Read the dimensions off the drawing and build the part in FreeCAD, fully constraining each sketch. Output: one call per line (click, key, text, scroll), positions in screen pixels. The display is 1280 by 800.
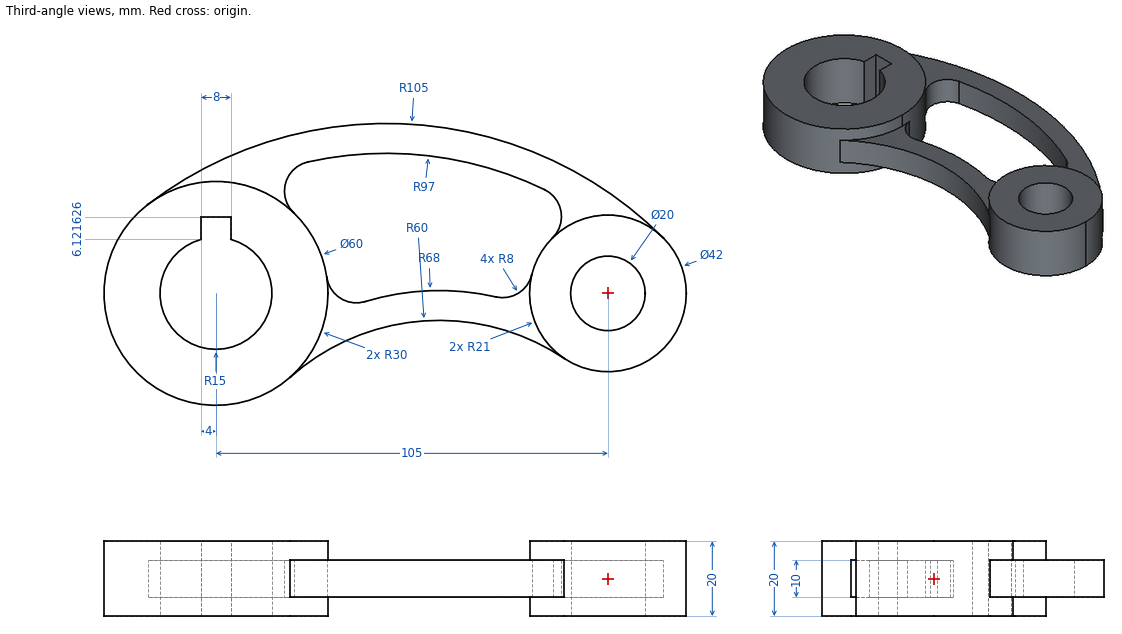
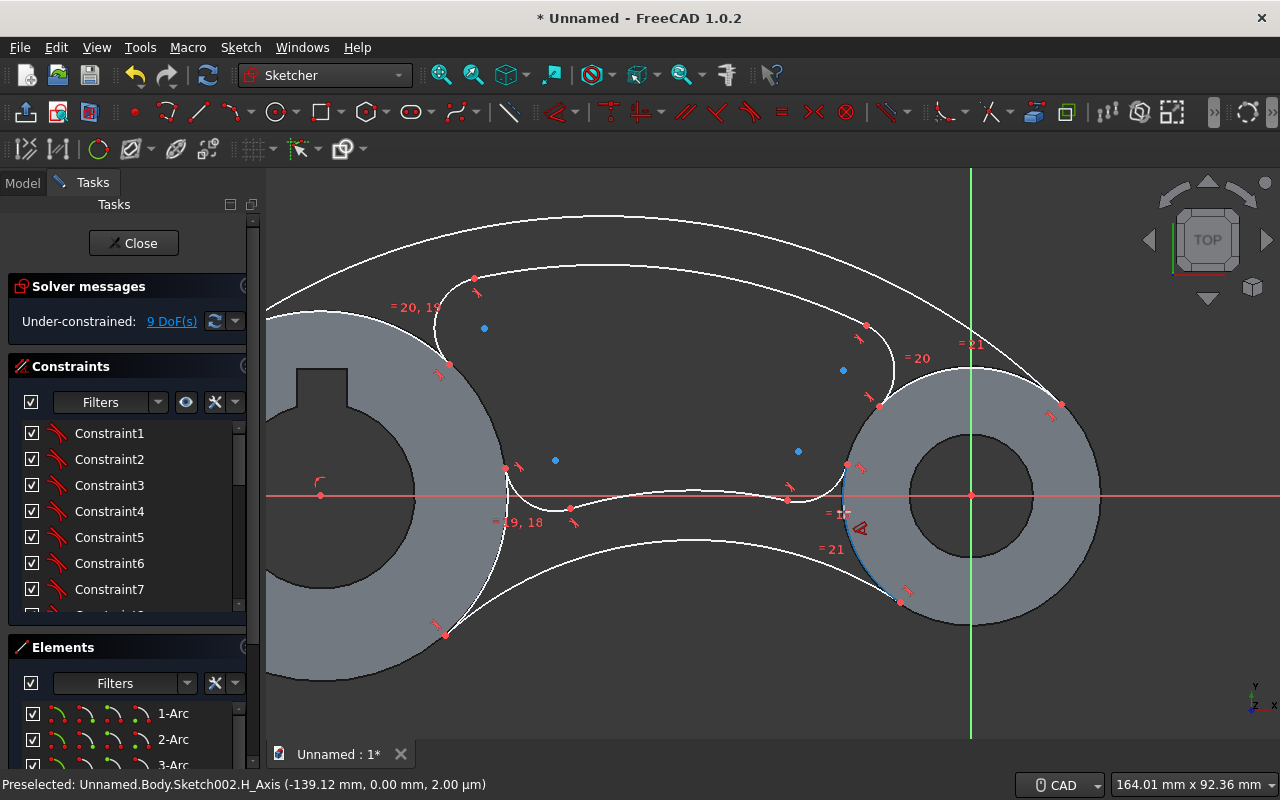
click(844, 511)
click(812, 515)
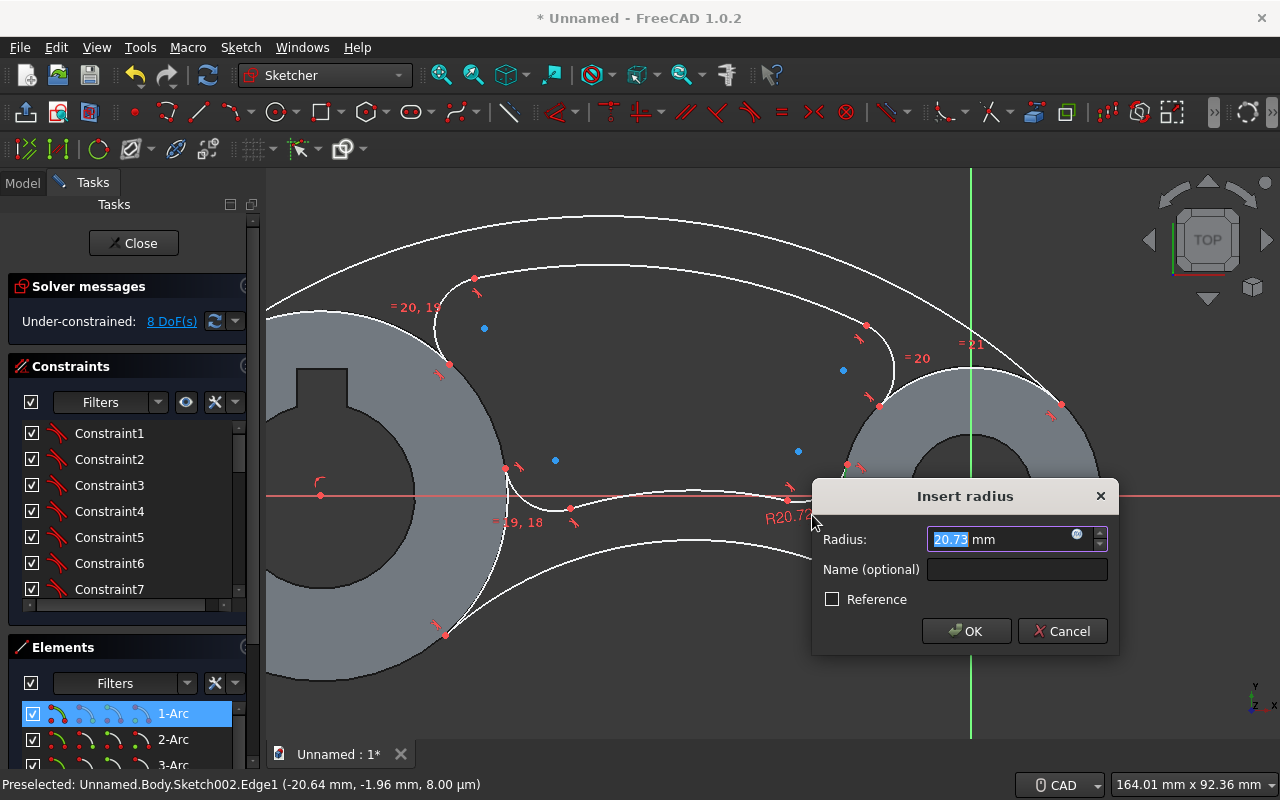
text(21)
key(Return)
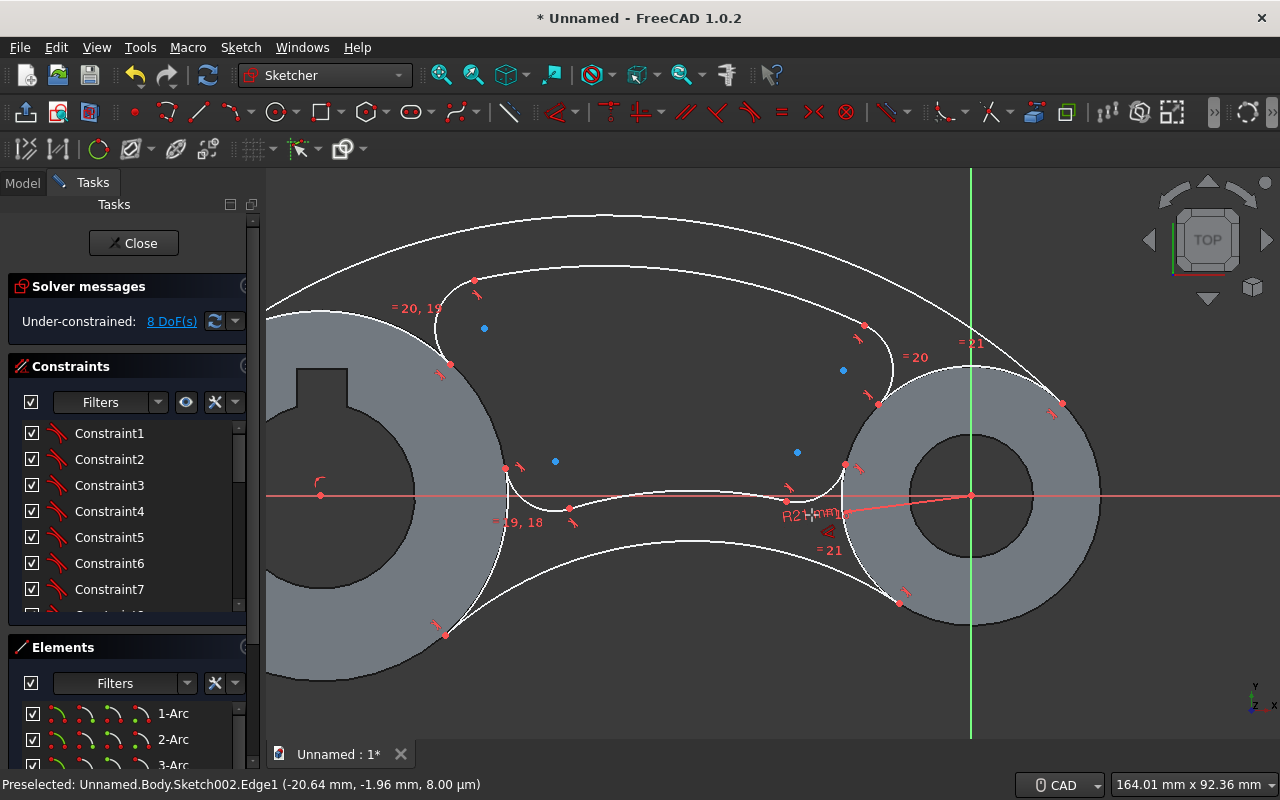
click(823, 495)
click(879, 454)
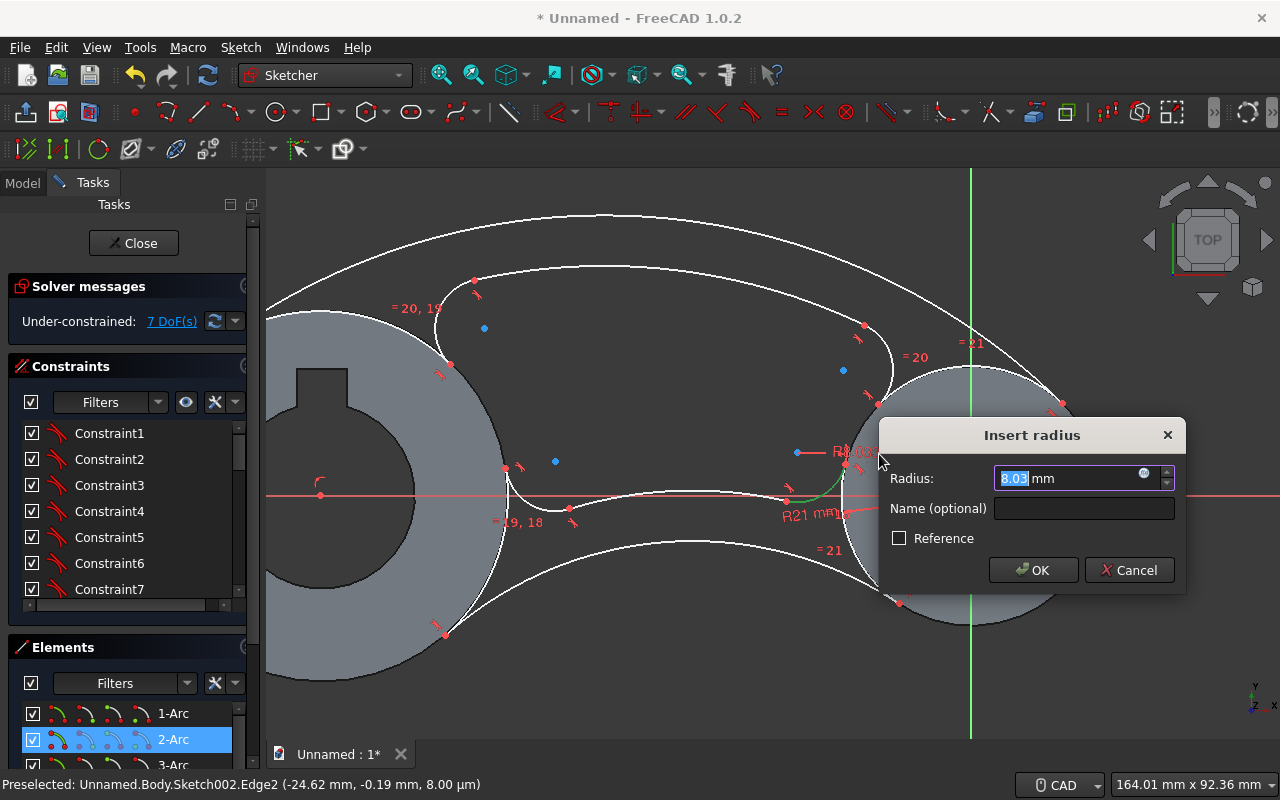
text(8)
key(Return)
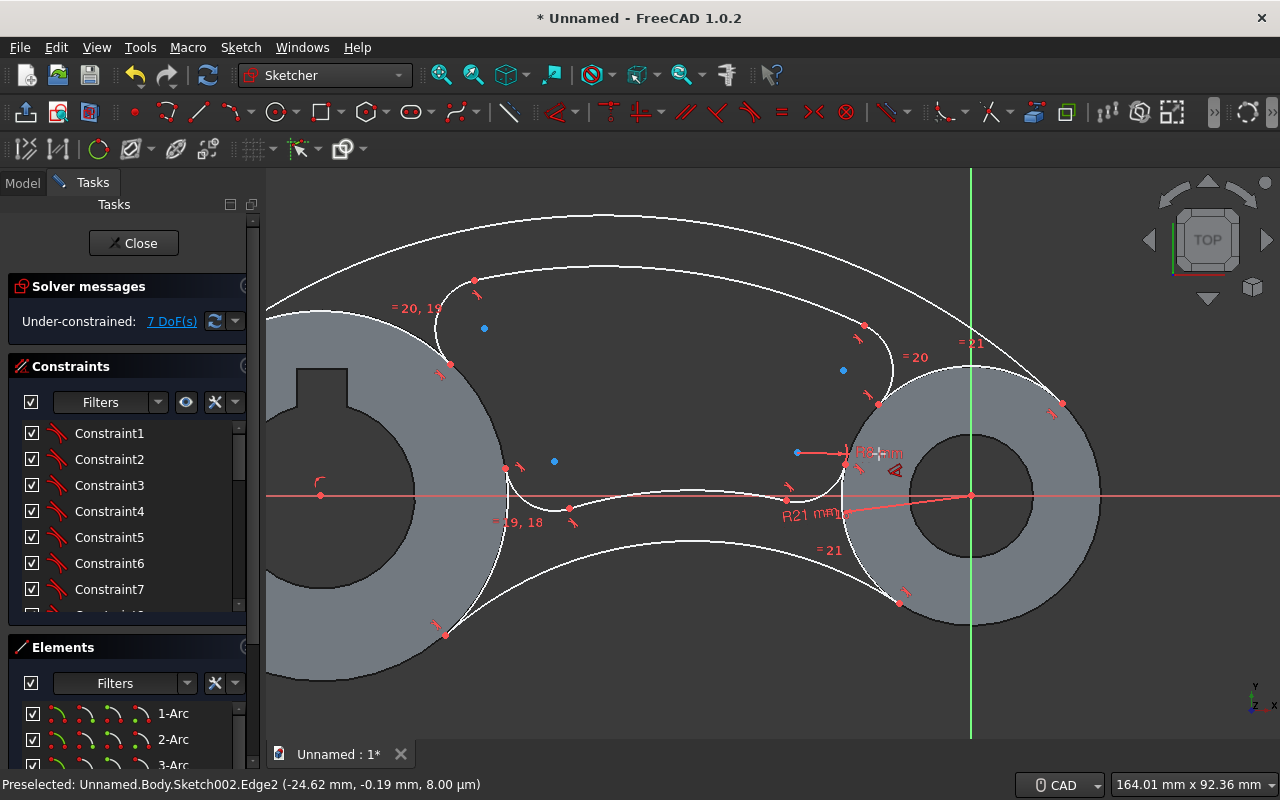
click(634, 494)
click(630, 462)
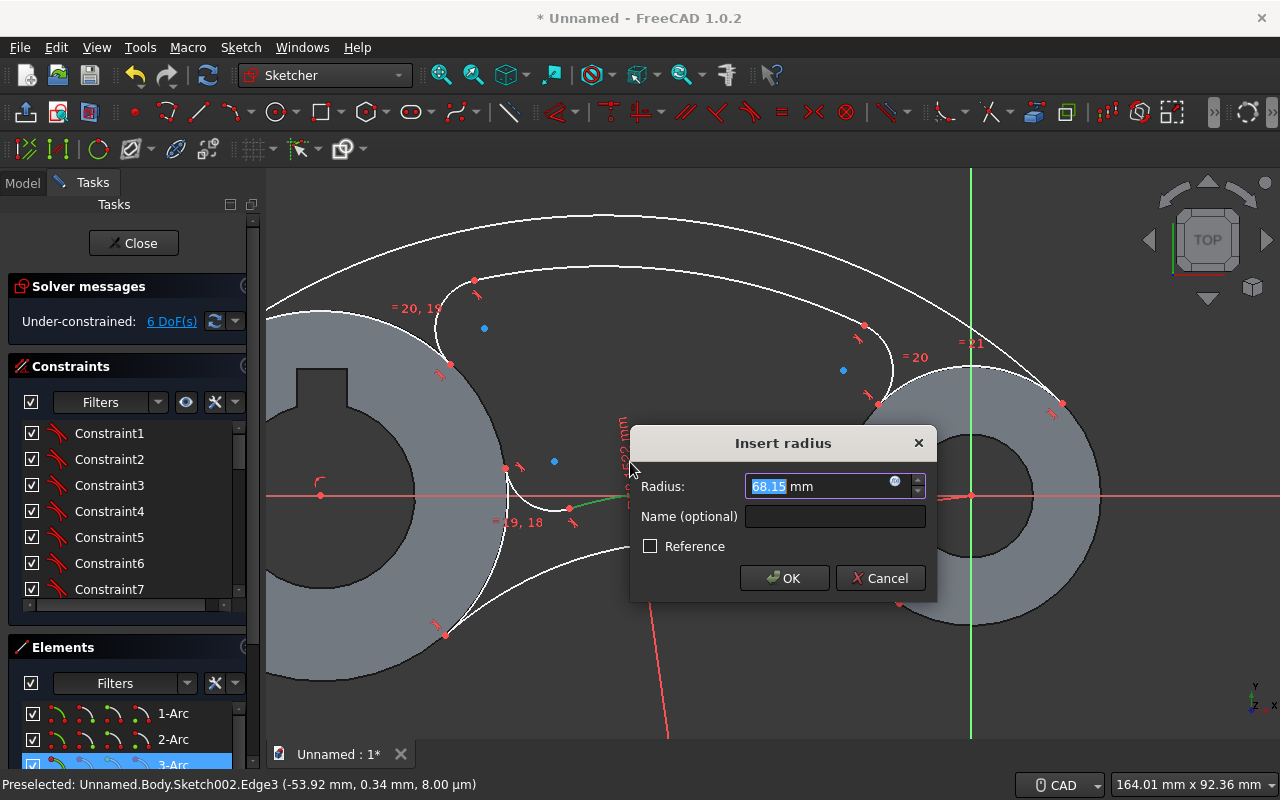
text(68)
key(Return)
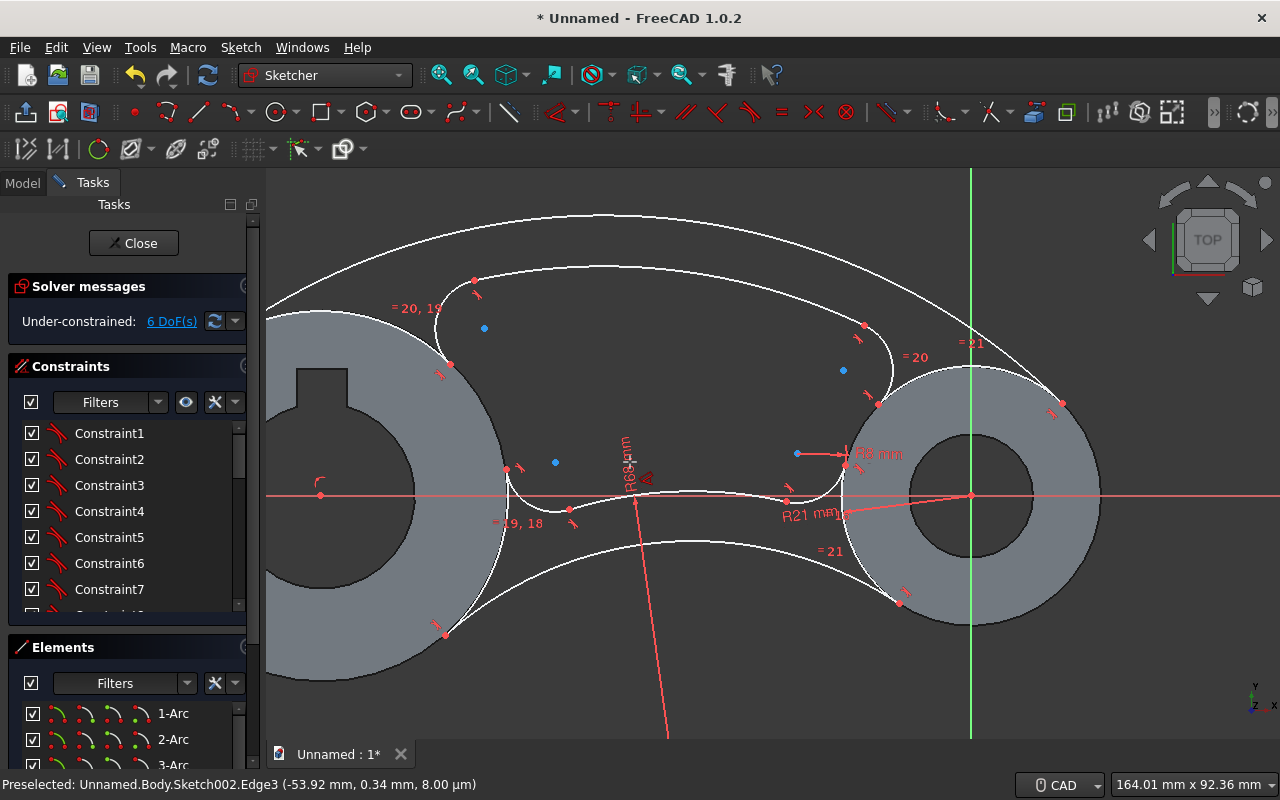
click(481, 593)
click(508, 610)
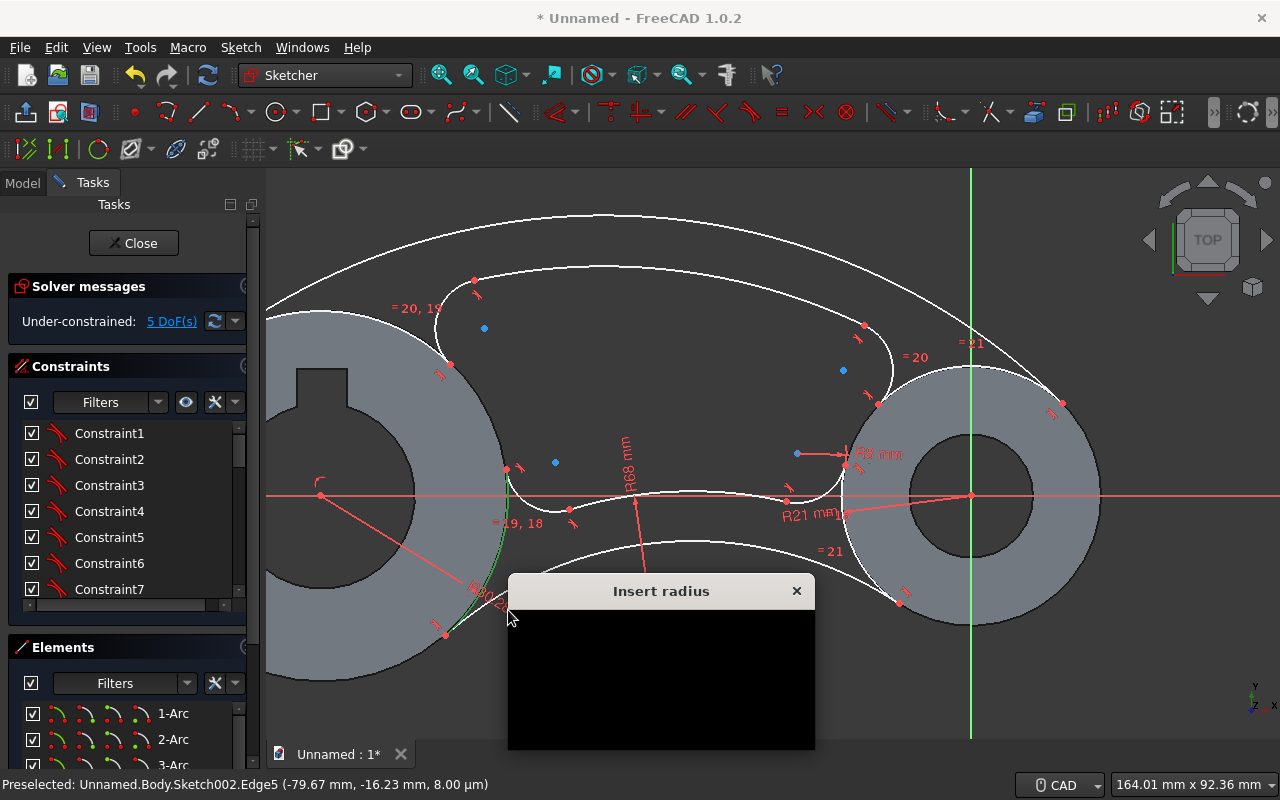
text(30)
key(Return)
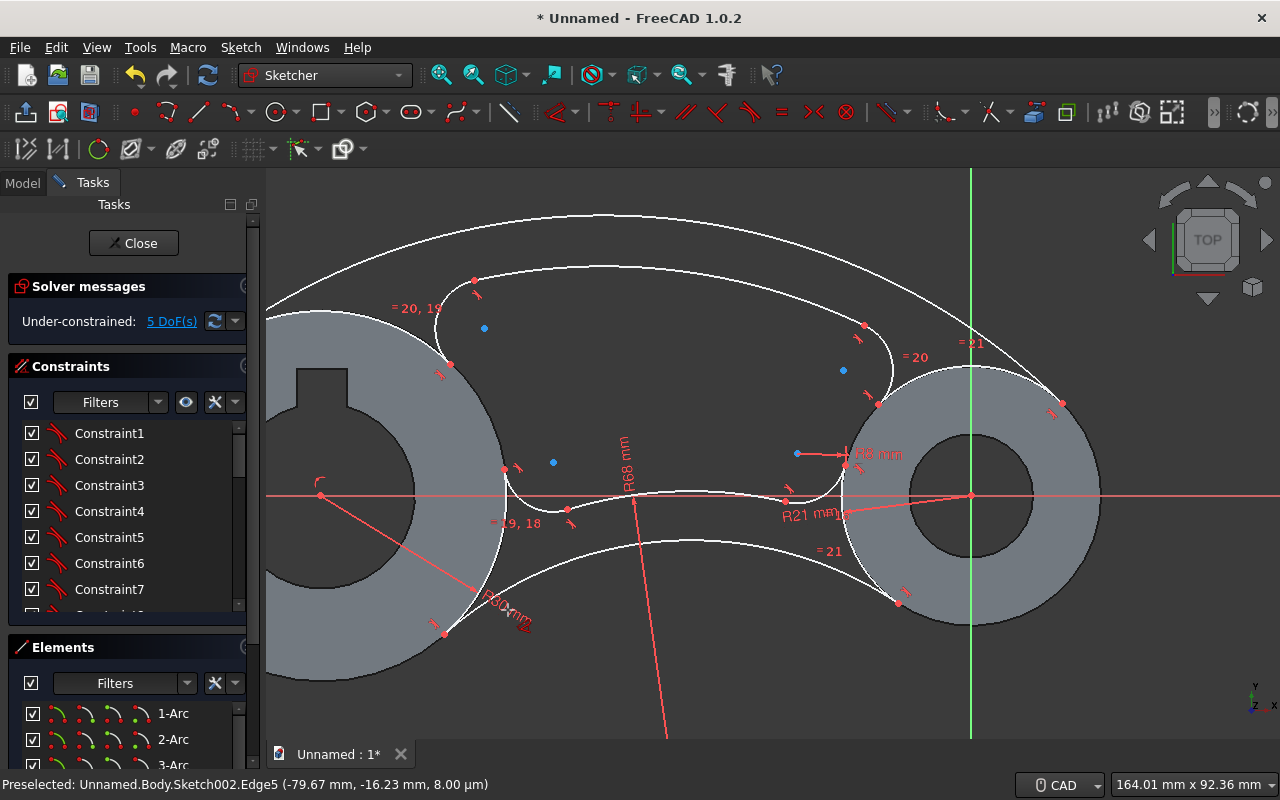
click(764, 547)
click(950, 602)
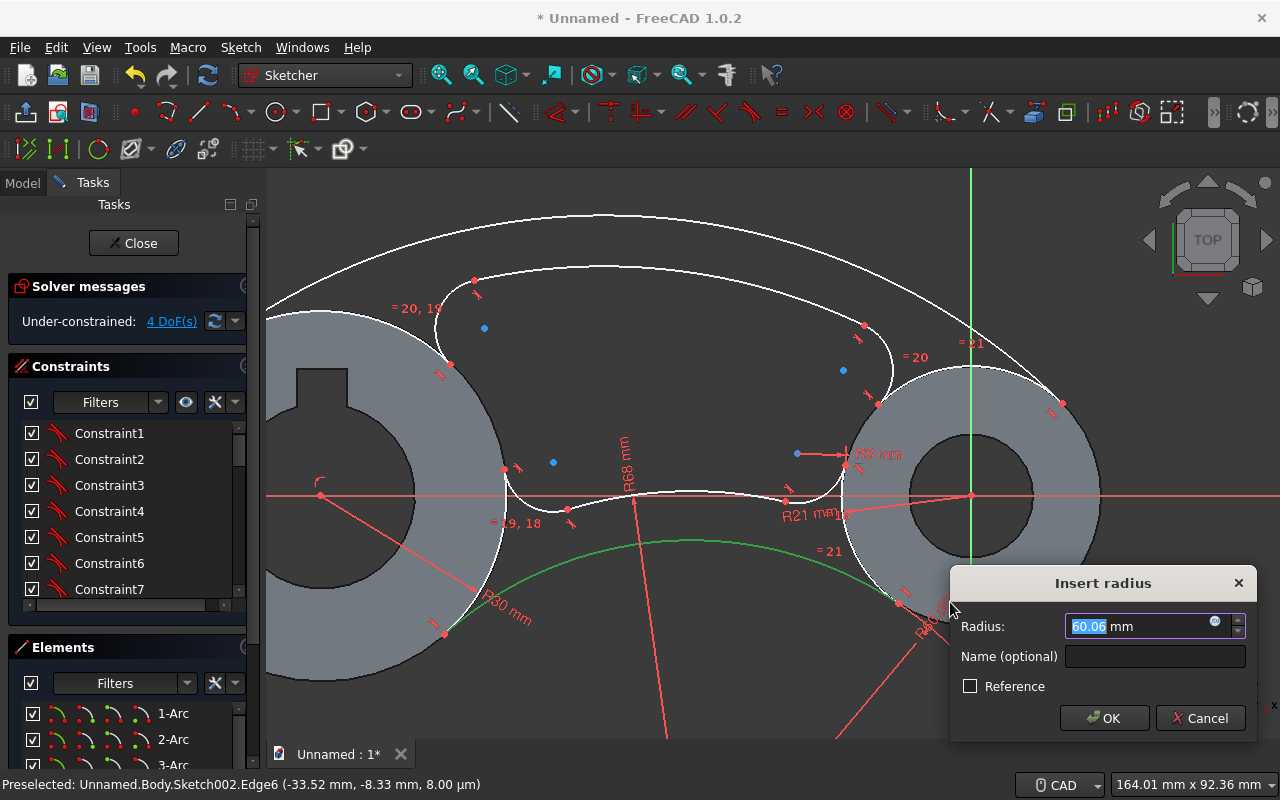
text(60)
key(Return)